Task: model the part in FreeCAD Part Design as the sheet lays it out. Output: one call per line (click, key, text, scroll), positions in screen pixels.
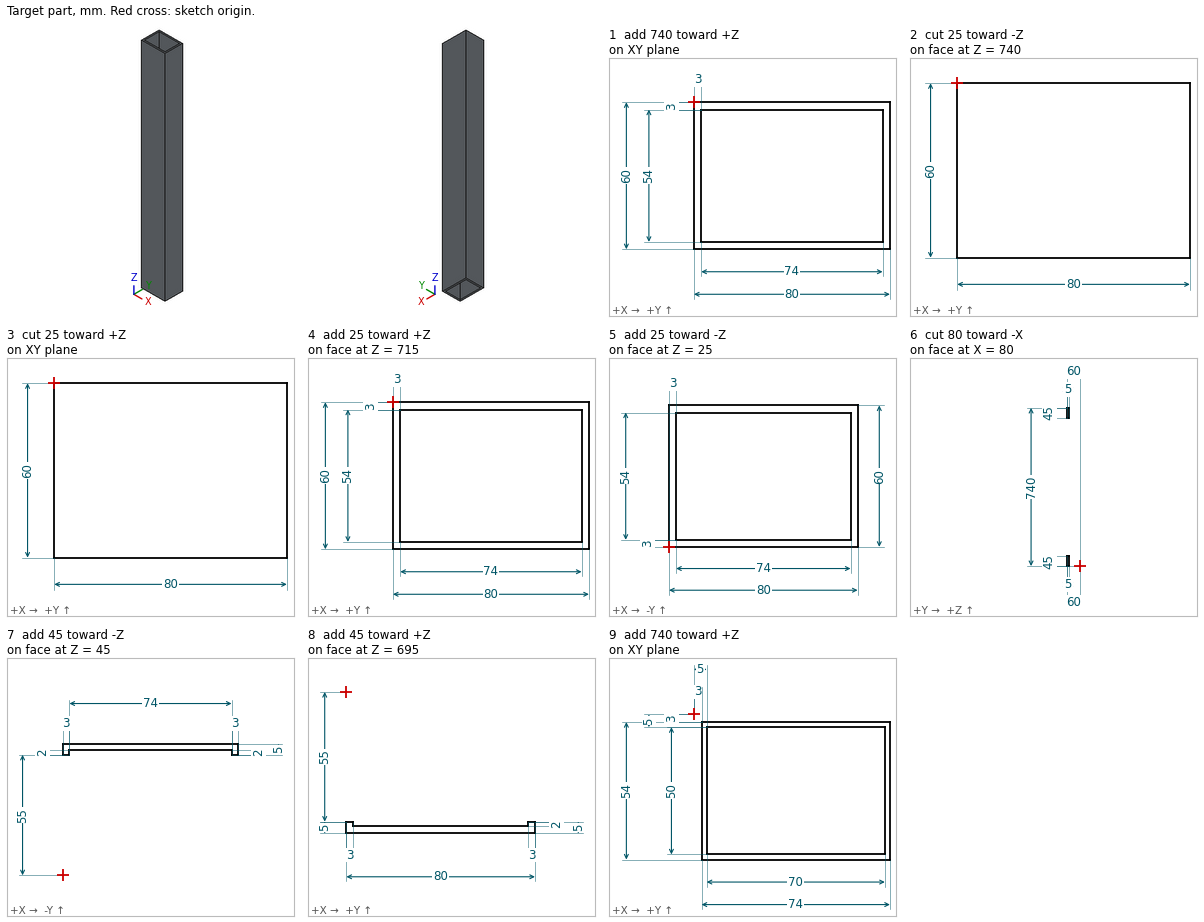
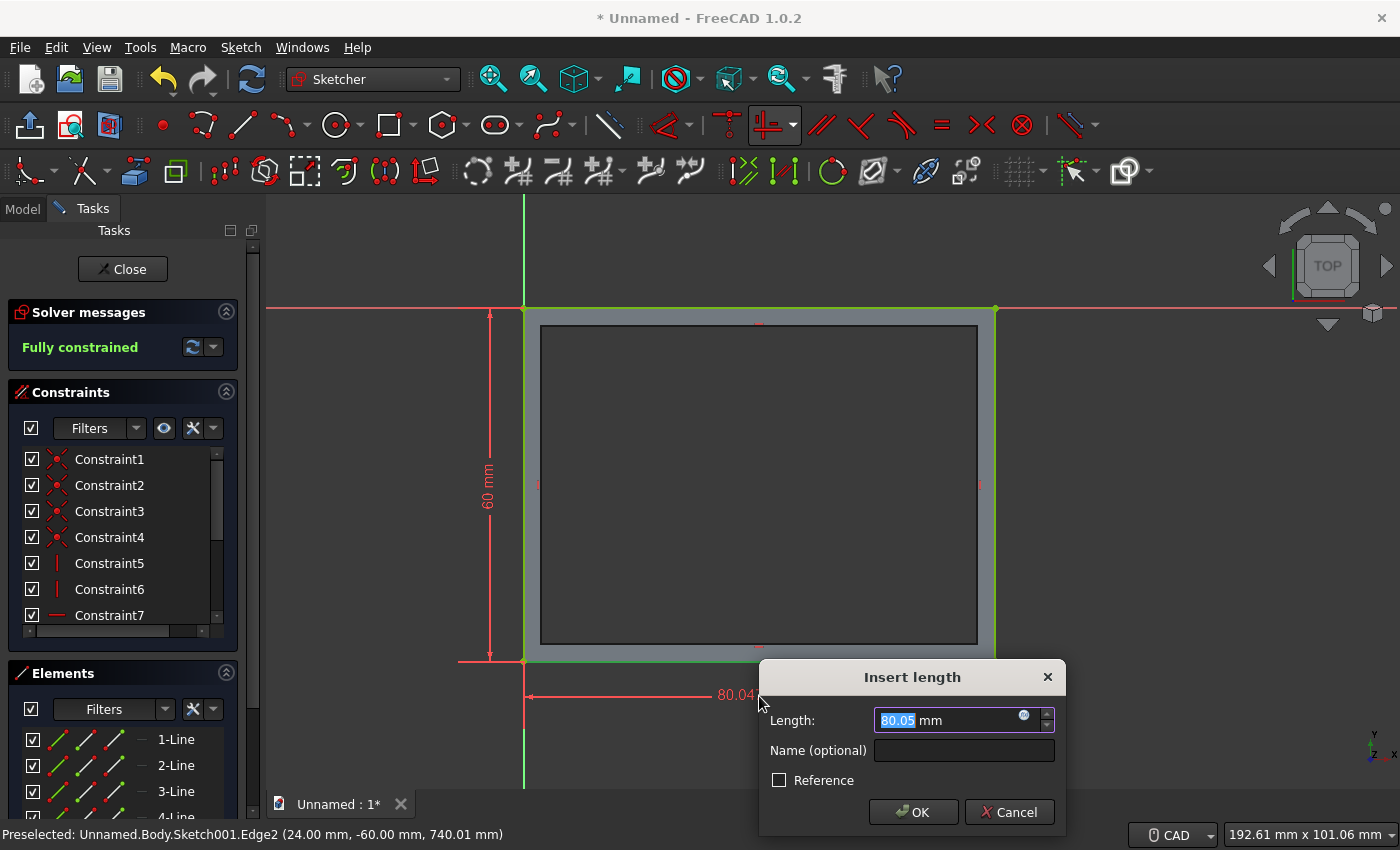
text(80)
key(Return)
key(Escape)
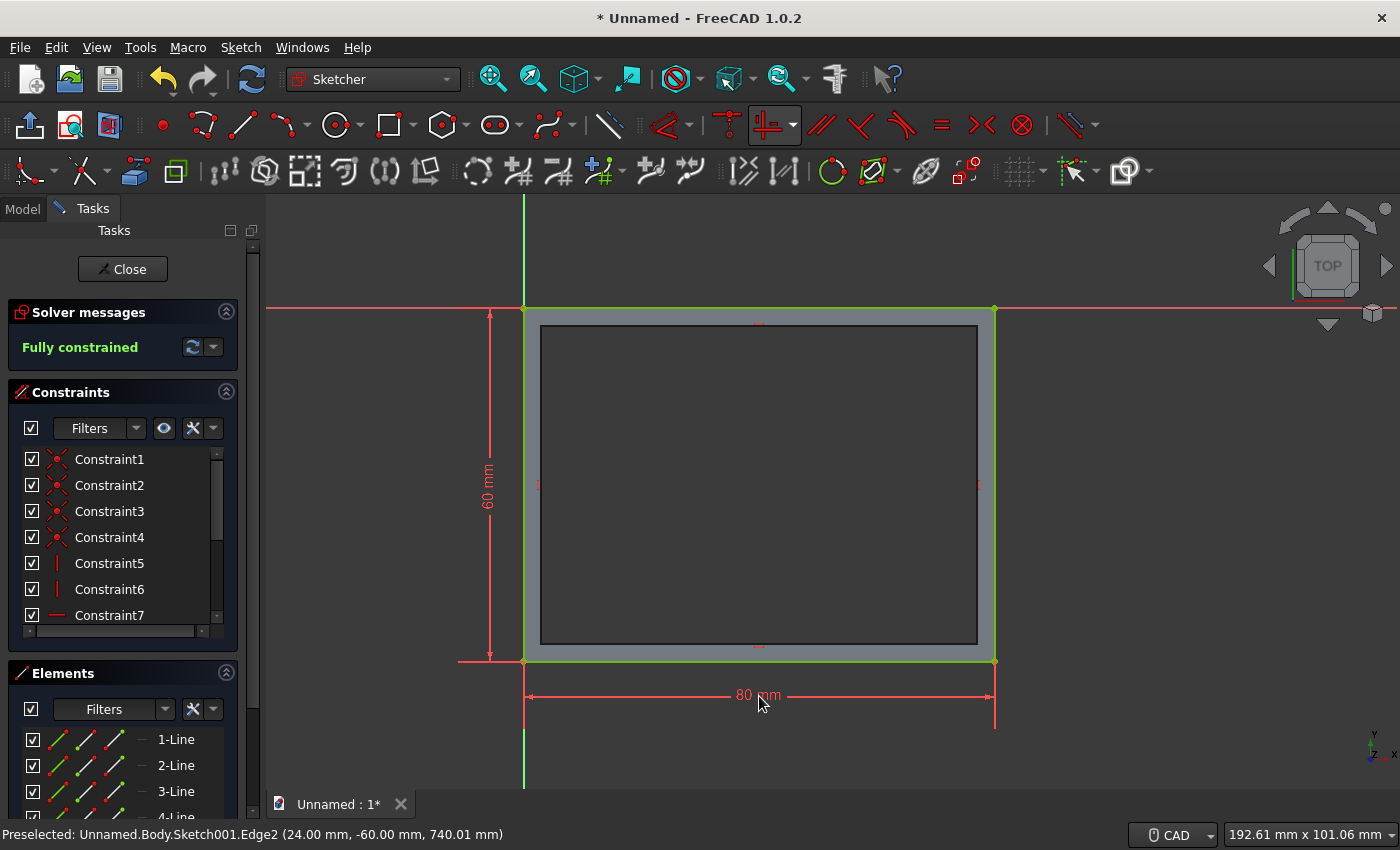
click(123, 269)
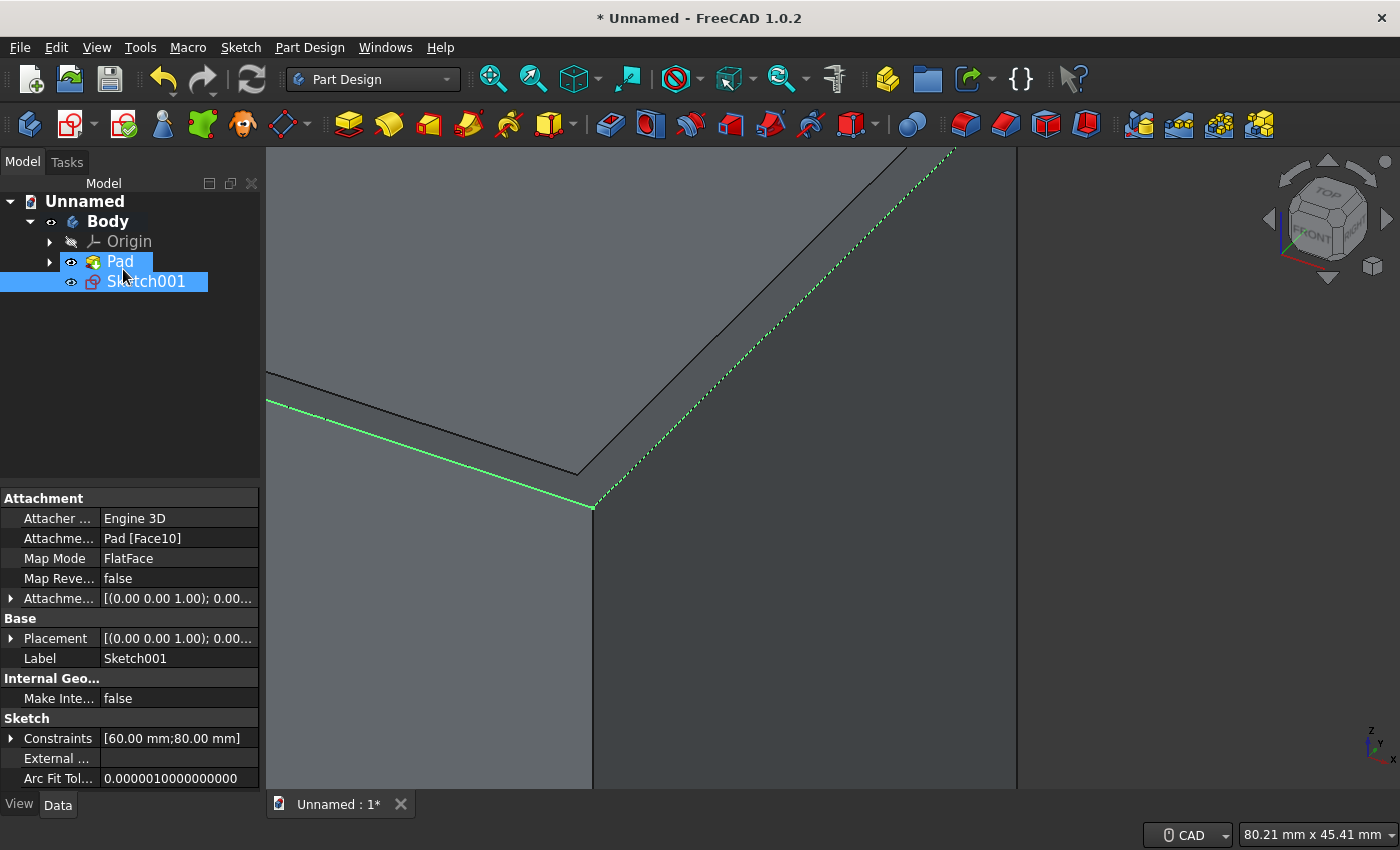
click(612, 124)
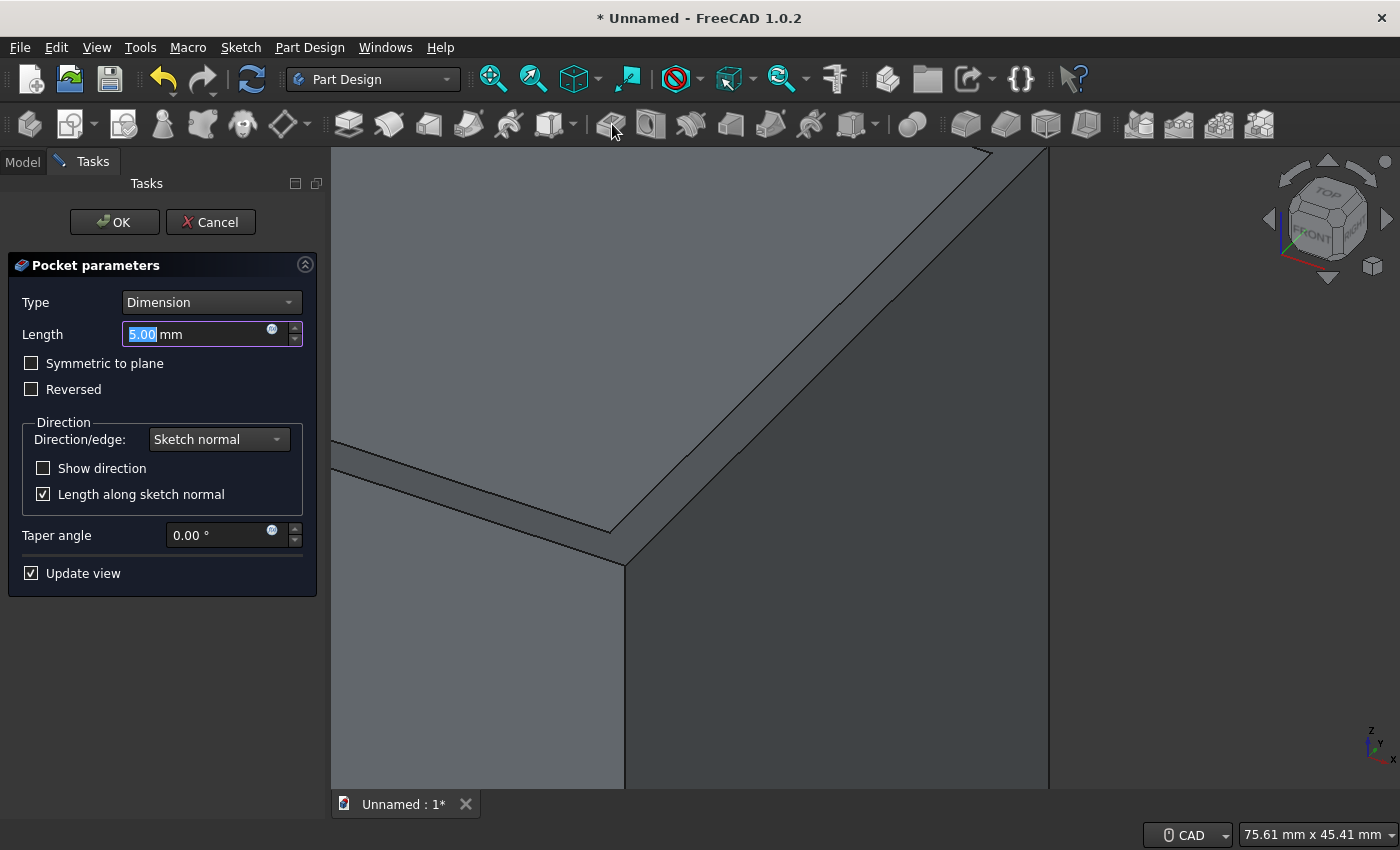
text(25)
key(Tab)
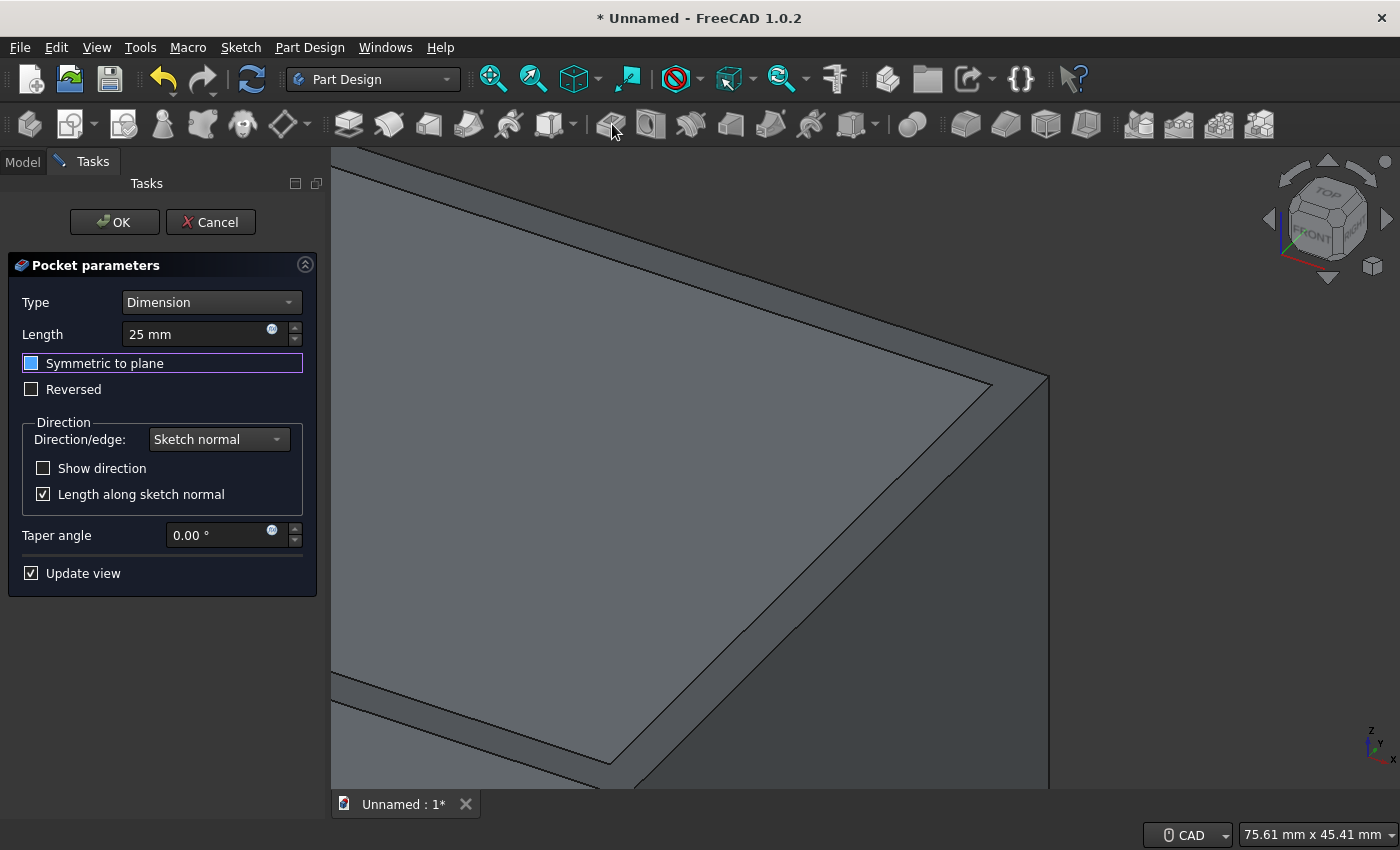
click(115, 222)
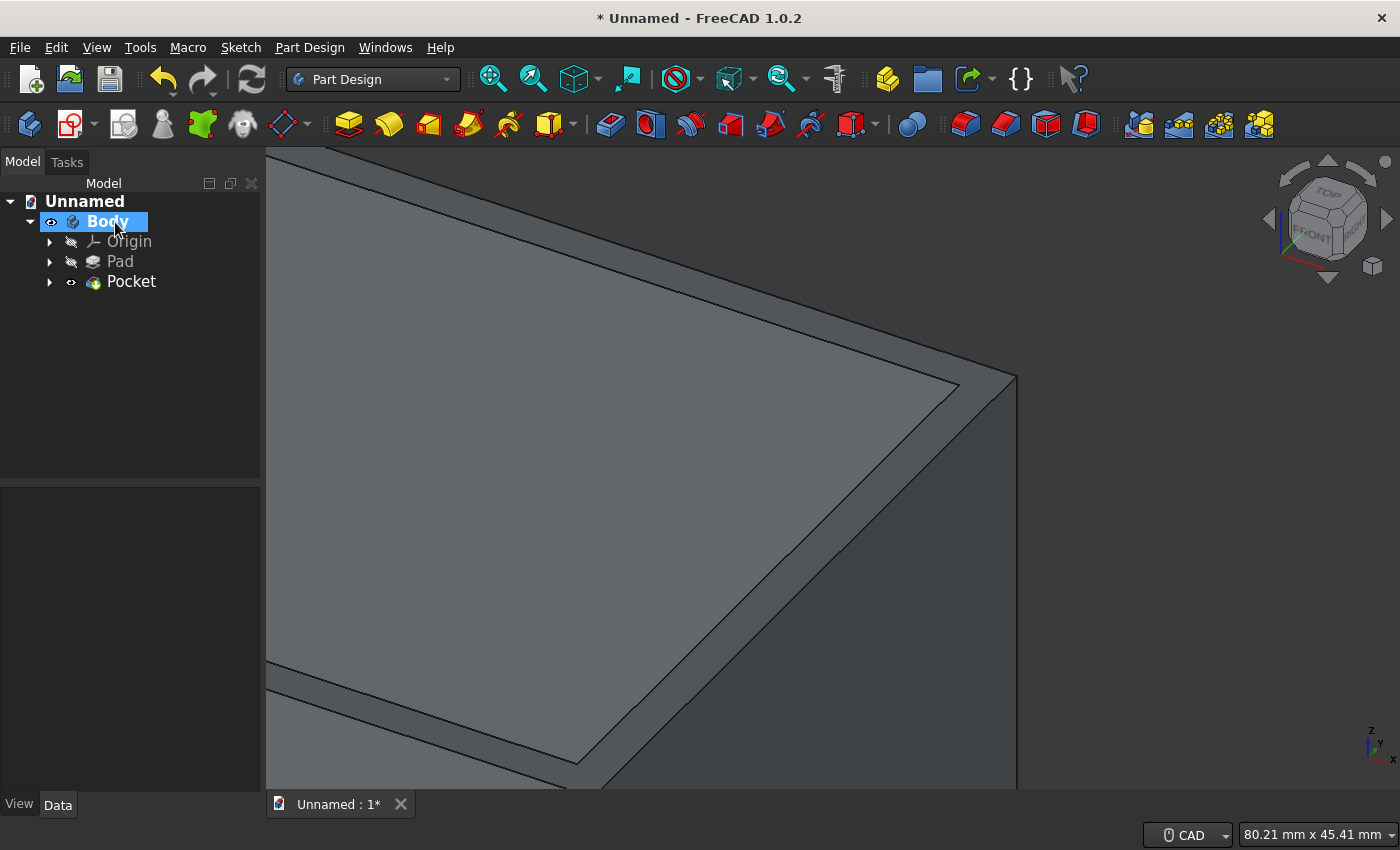
key(v)
key(f)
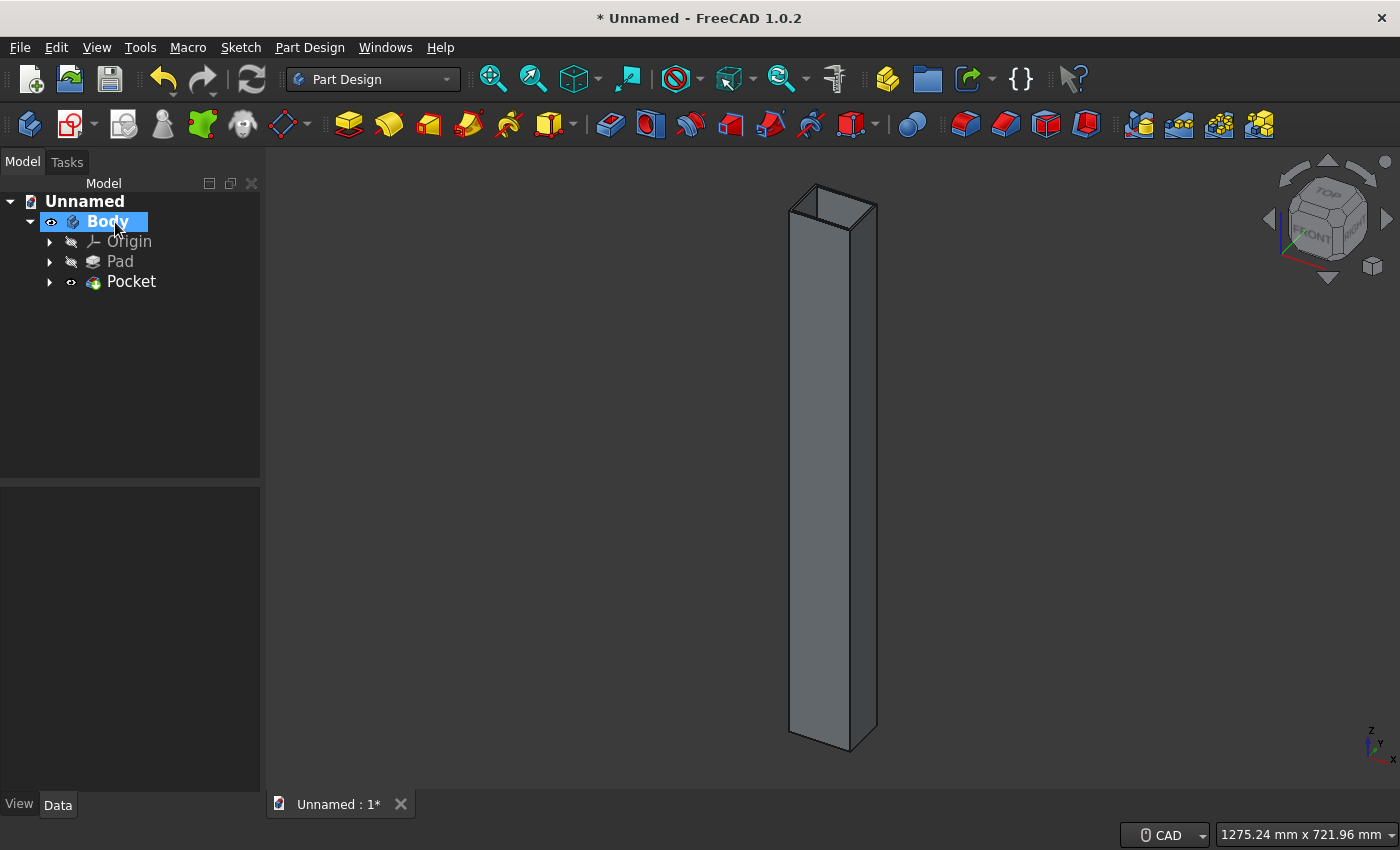
click(70, 124)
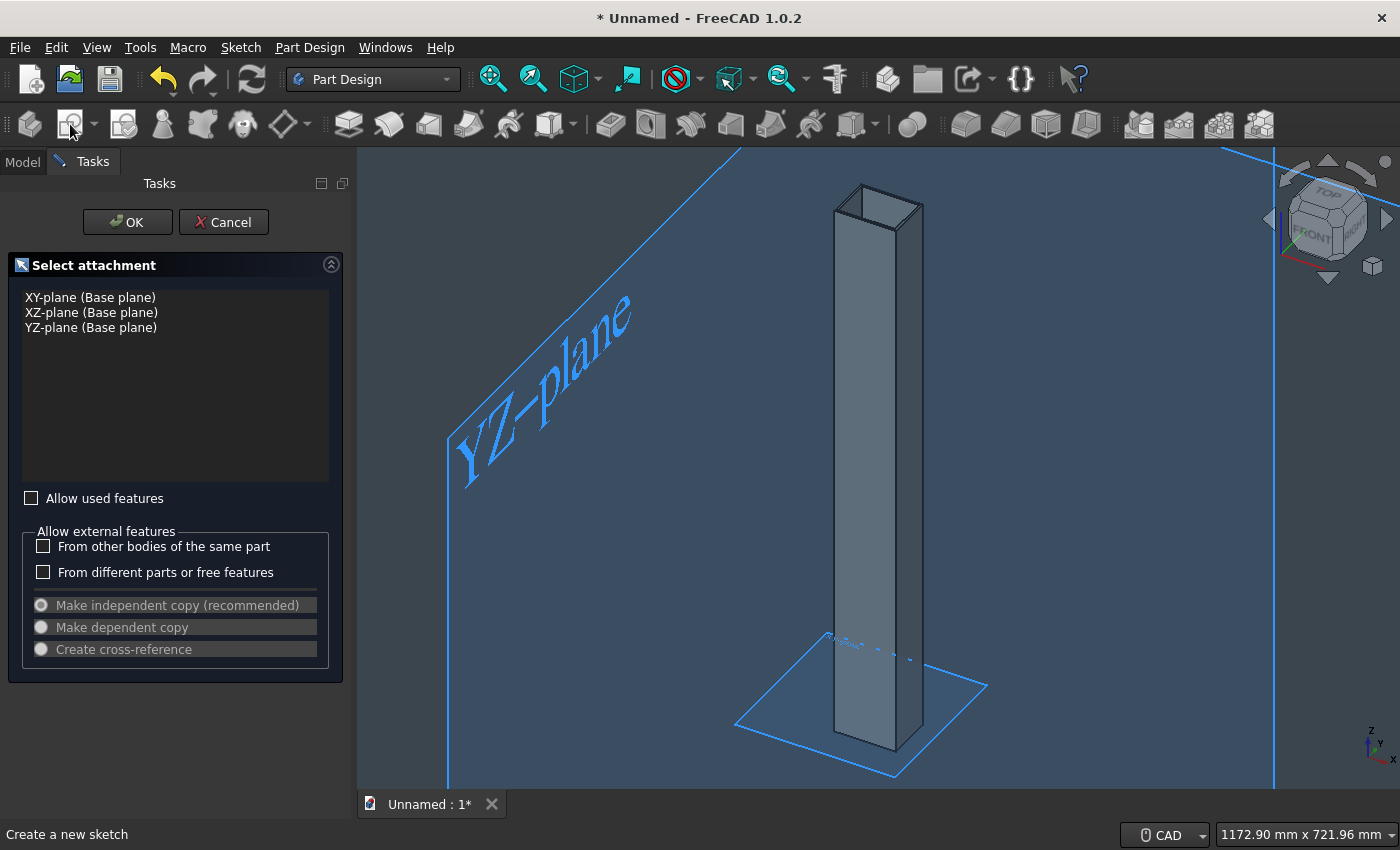
click(82, 298)